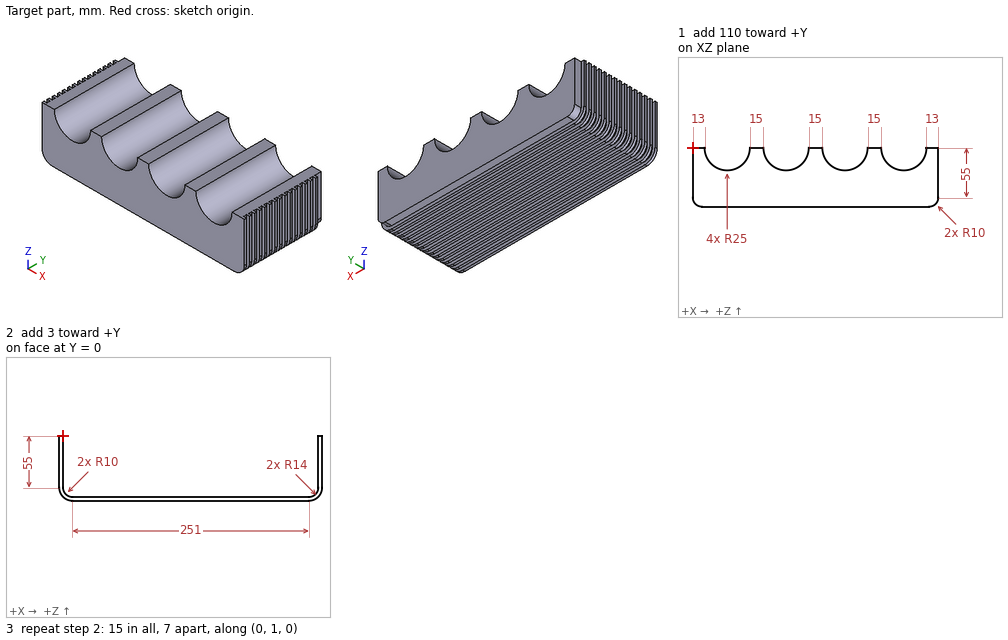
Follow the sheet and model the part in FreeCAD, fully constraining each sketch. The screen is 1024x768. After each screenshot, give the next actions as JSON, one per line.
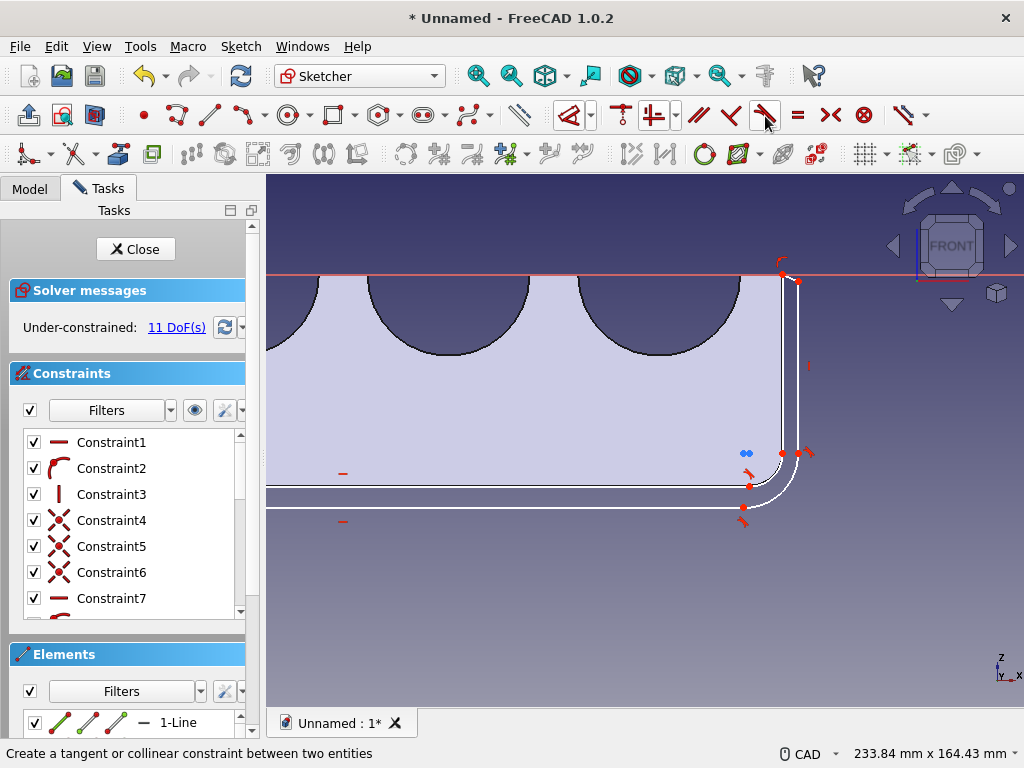
{"action": "scroll", "coordinate": [767, 484], "scroll_direction": "down", "scroll_amount": 4}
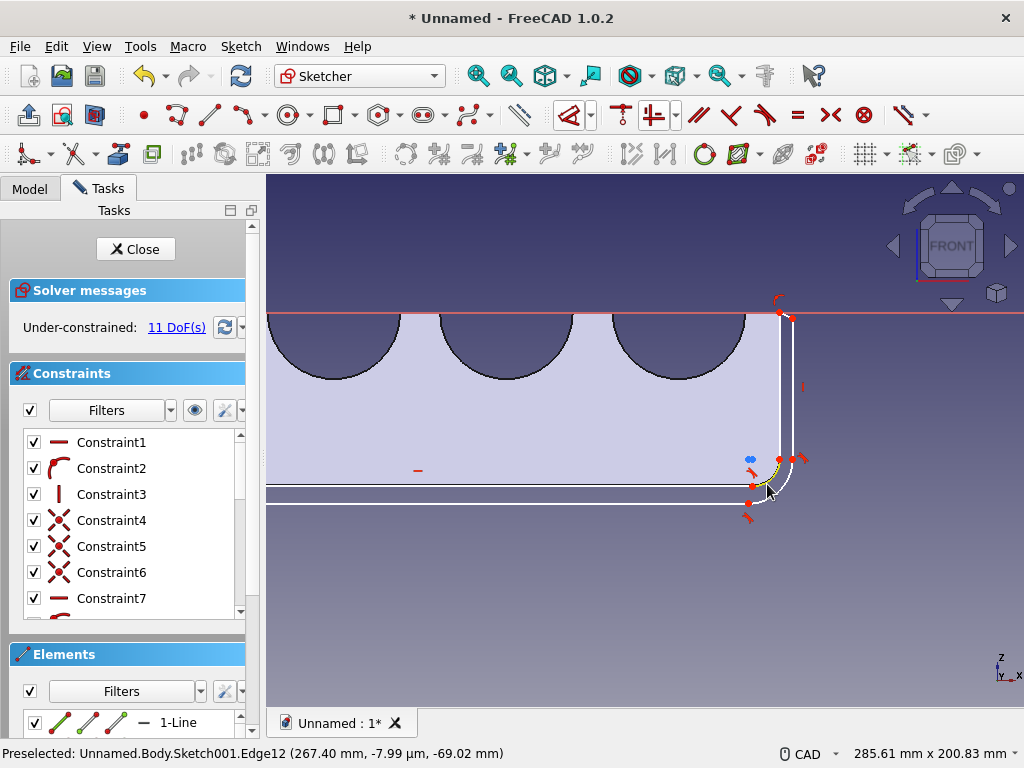
{"action": "scroll", "coordinate": [380, 414], "scroll_direction": "up", "scroll_amount": 5}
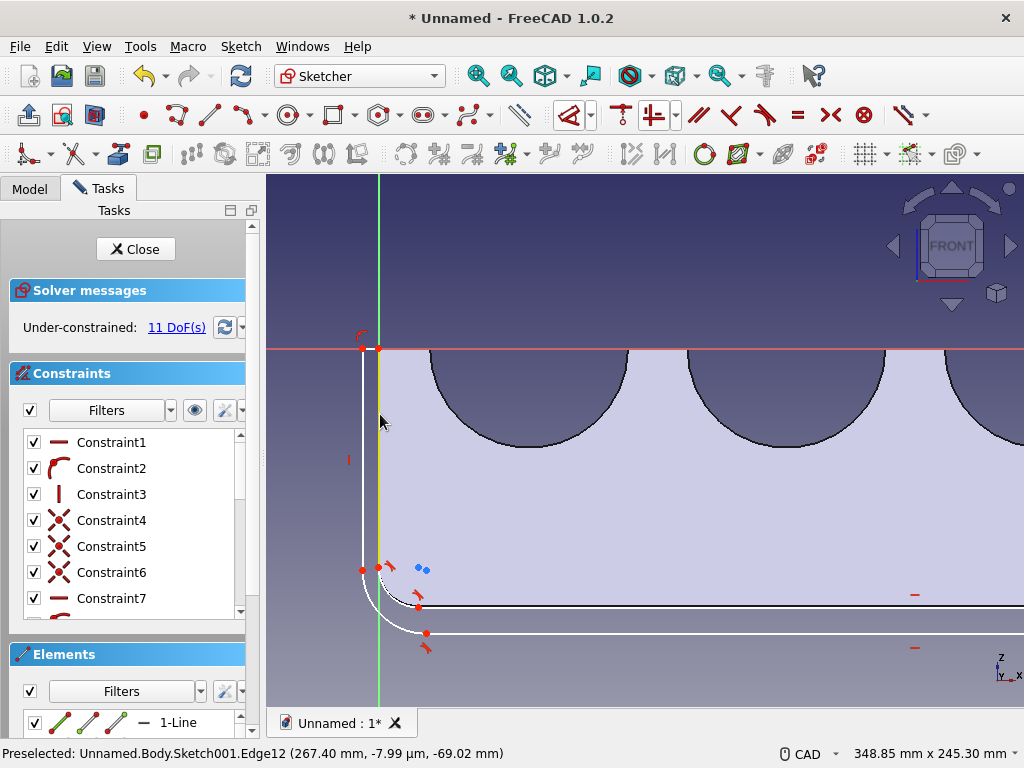
{"action": "left_click", "coordinate": [379, 414]}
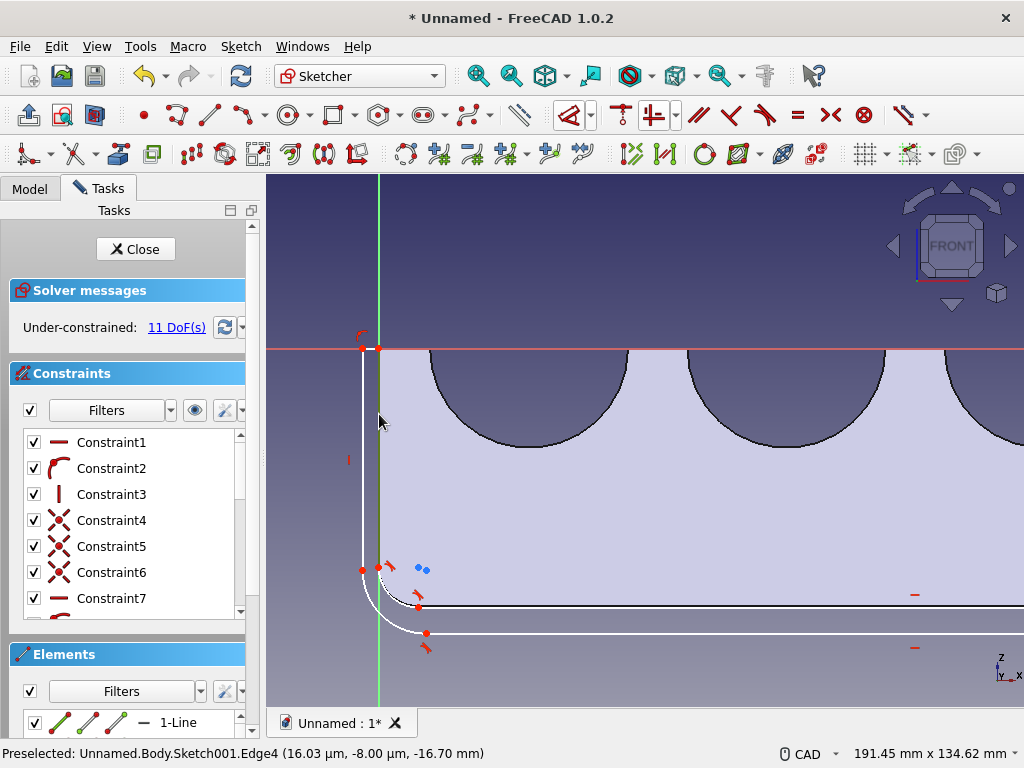
{"action": "key", "text": "v"}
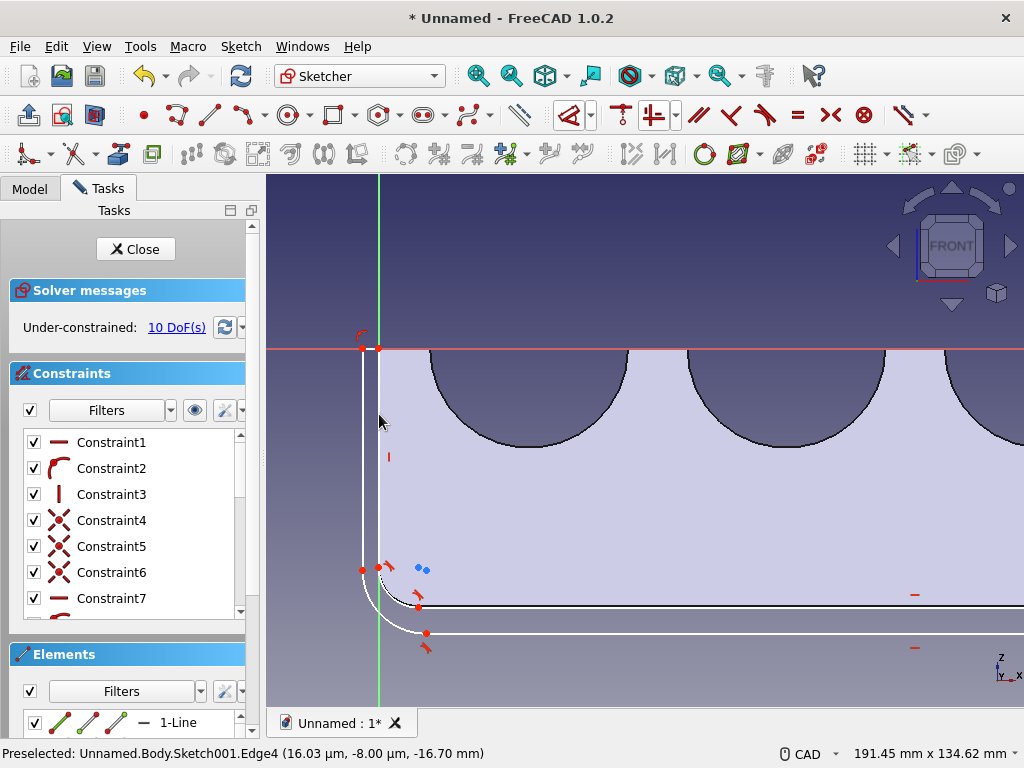
{"action": "scroll", "coordinate": [379, 414], "scroll_direction": "down", "scroll_amount": 5}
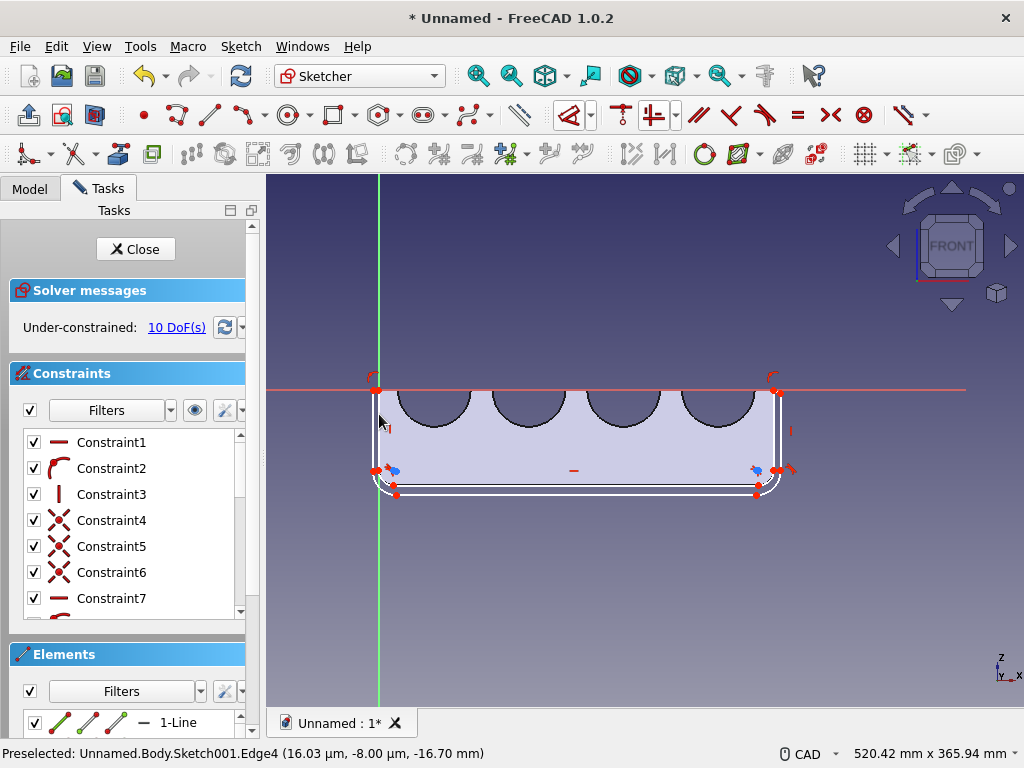
{"action": "scroll", "coordinate": [777, 392], "scroll_direction": "up", "scroll_amount": 9}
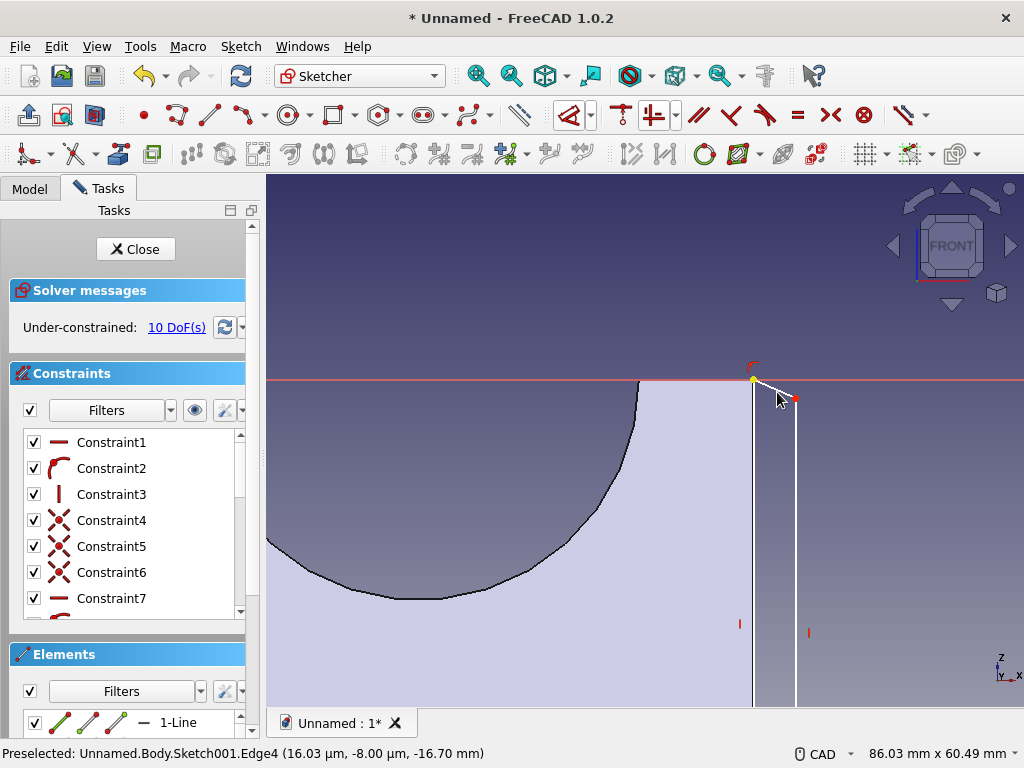
{"action": "left_click", "coordinate": [771, 387]}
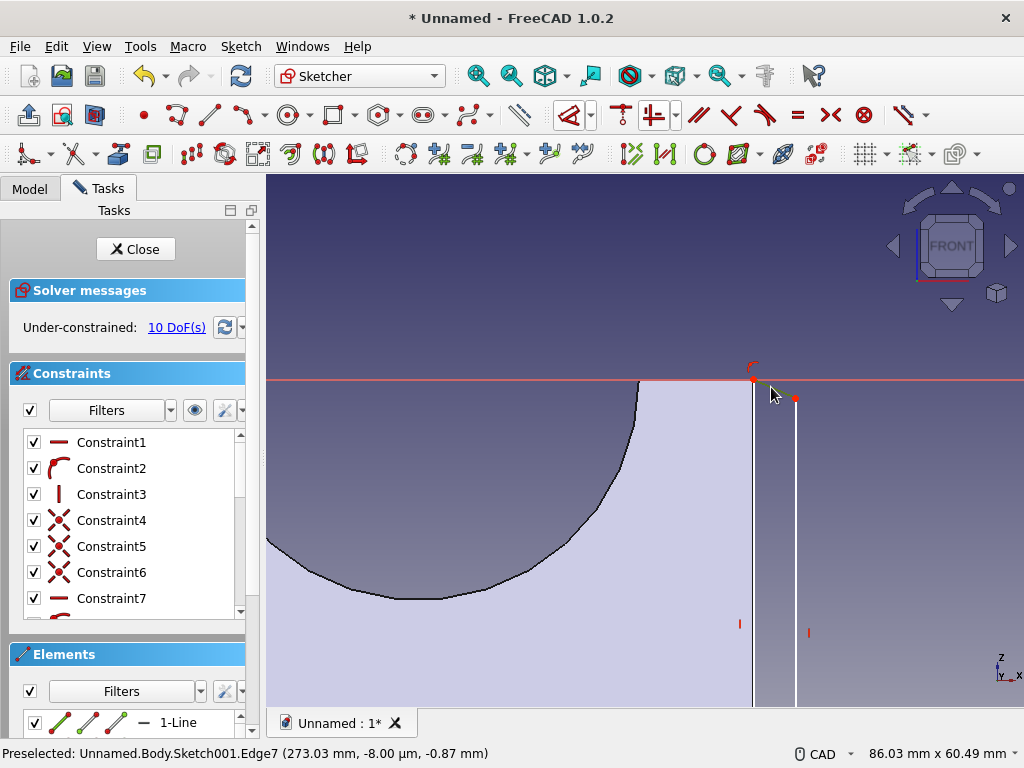
{"action": "key", "text": "h"}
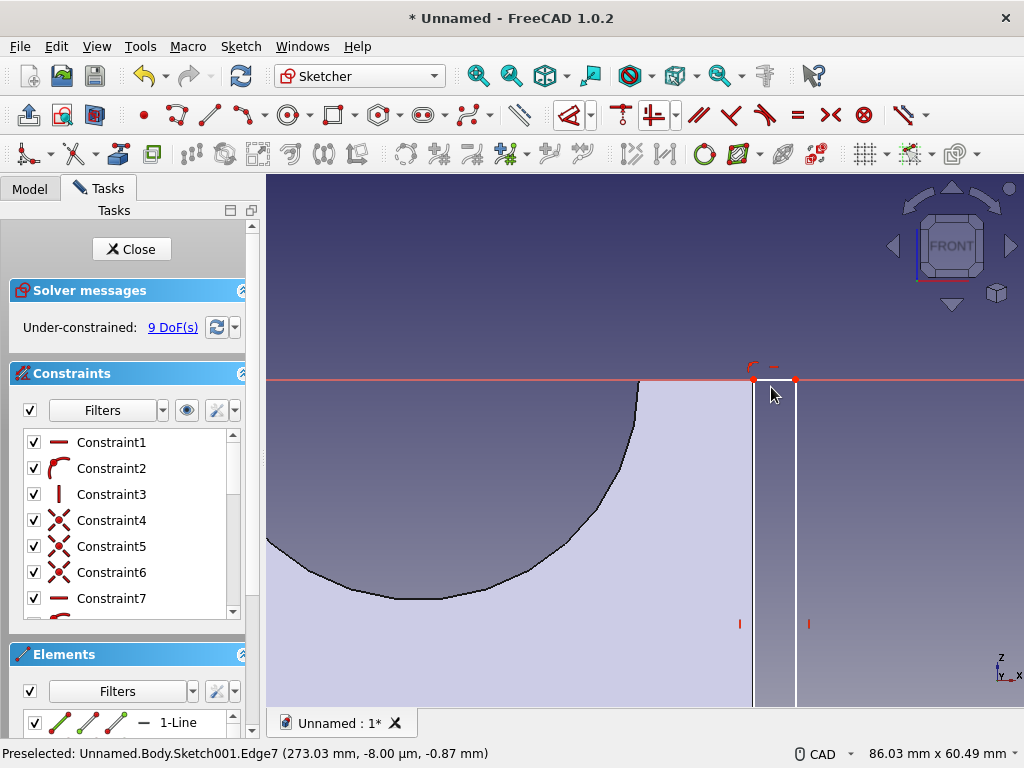
{"action": "scroll", "coordinate": [778, 392], "scroll_direction": "down", "scroll_amount": 9}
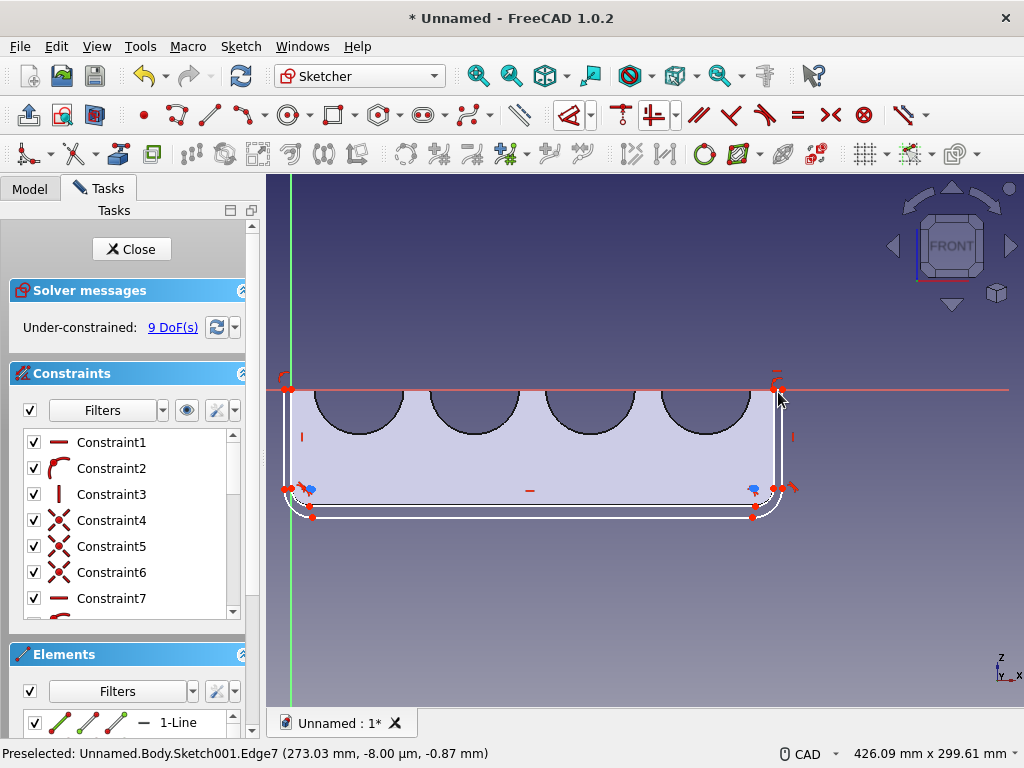
{"action": "scroll", "coordinate": [376, 482], "scroll_direction": "up", "scroll_amount": 8}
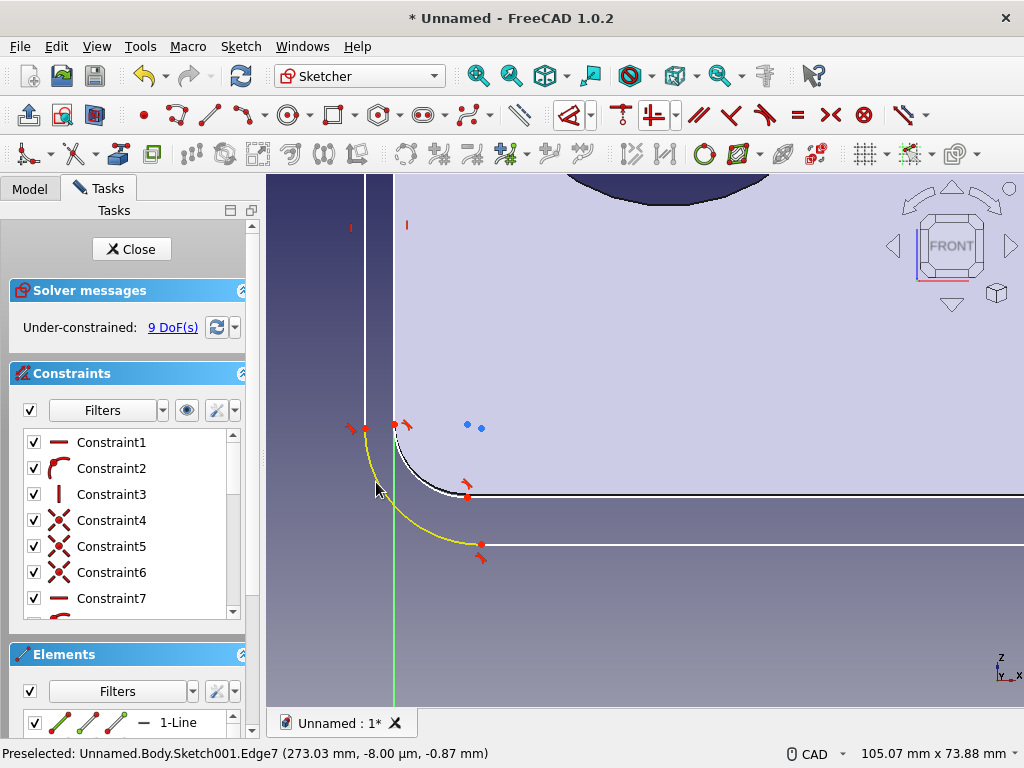
{"action": "left_click", "coordinate": [378, 481]}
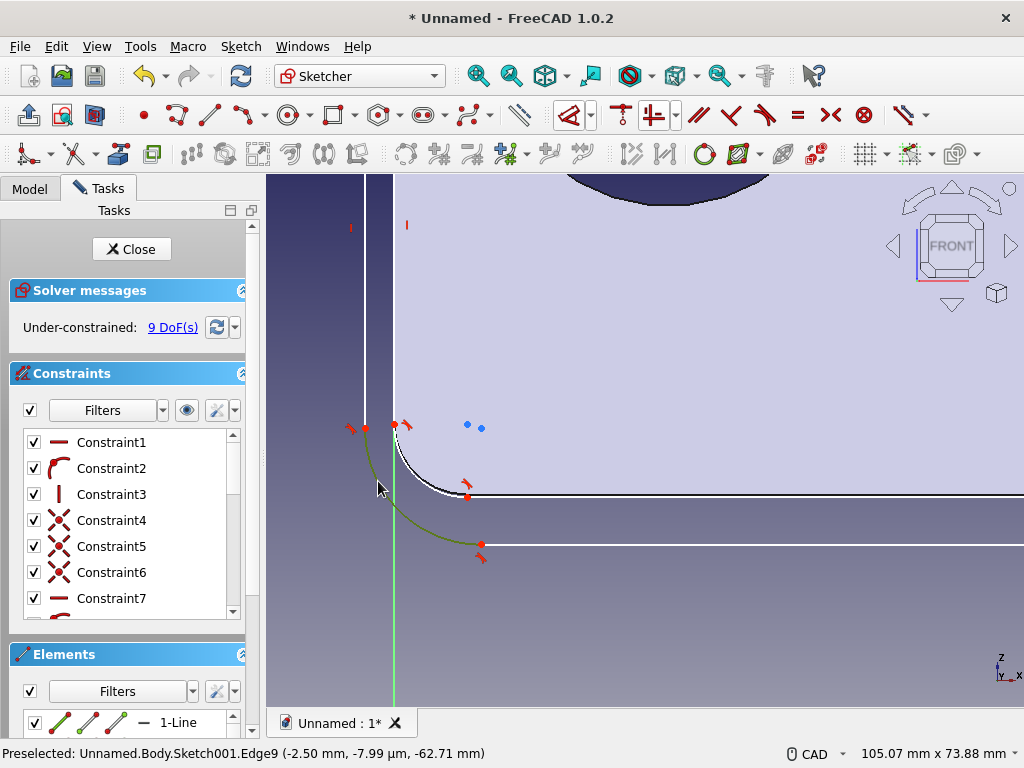
{"action": "left_click", "coordinate": [434, 489]}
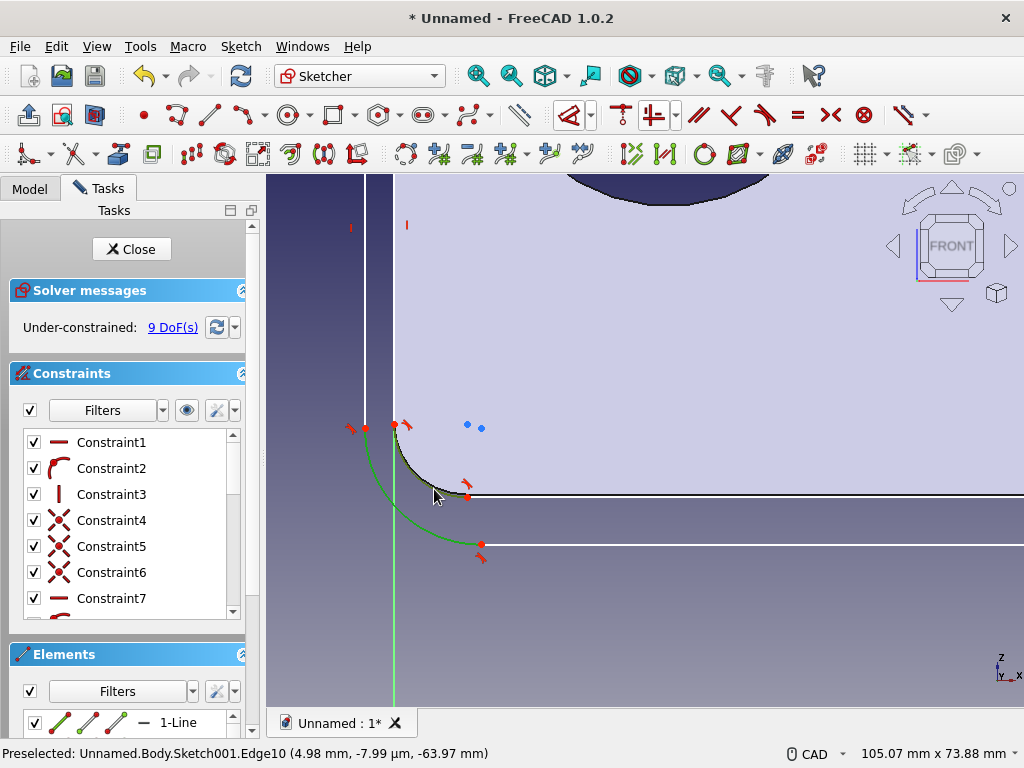
{"action": "key", "text": "c"}